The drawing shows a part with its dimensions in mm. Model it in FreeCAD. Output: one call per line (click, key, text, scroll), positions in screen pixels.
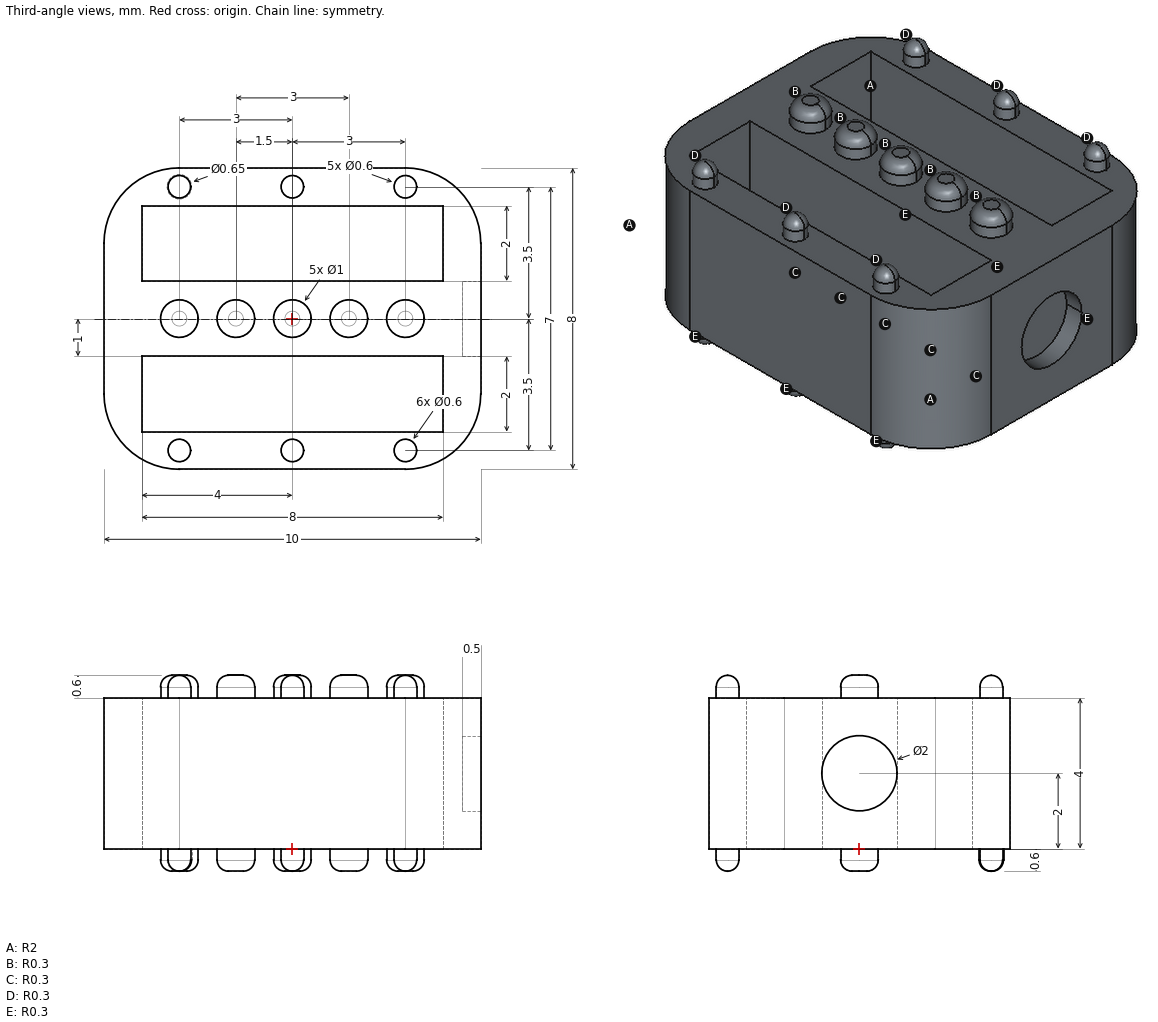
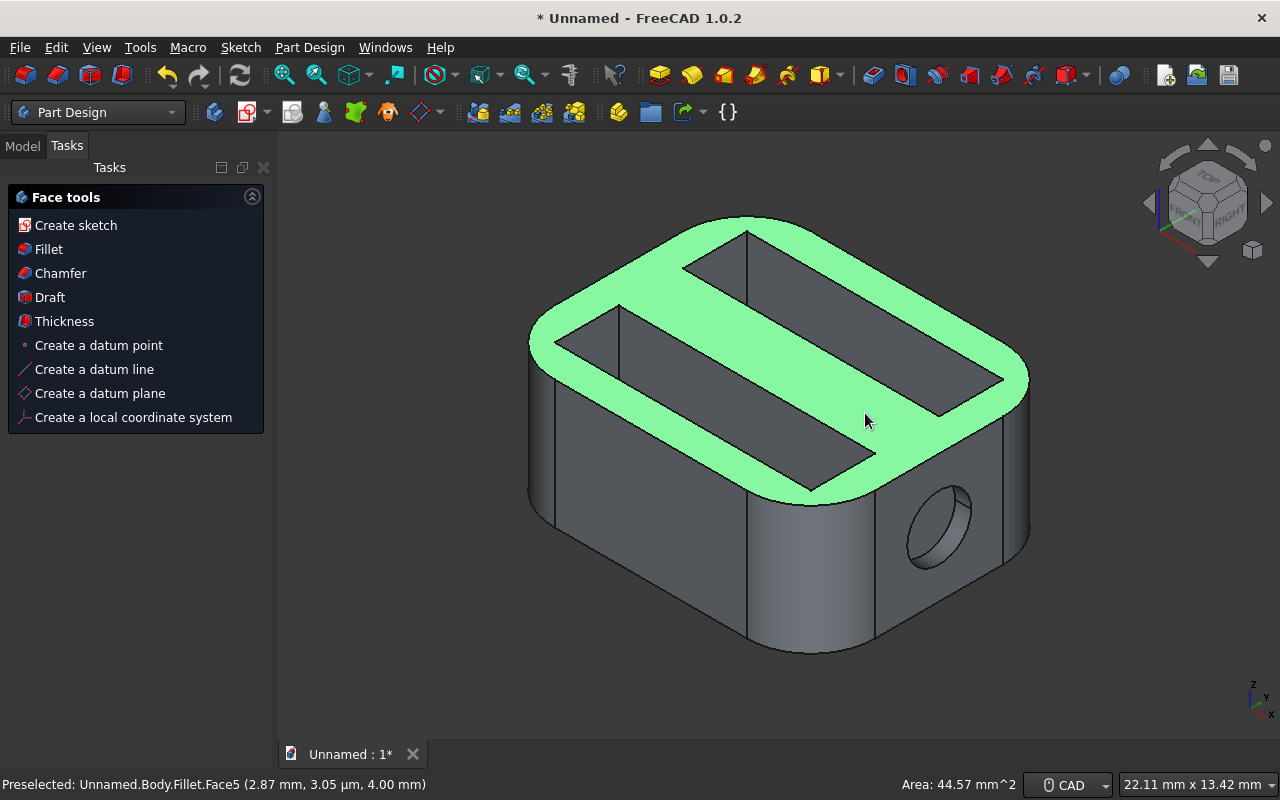
click(248, 112)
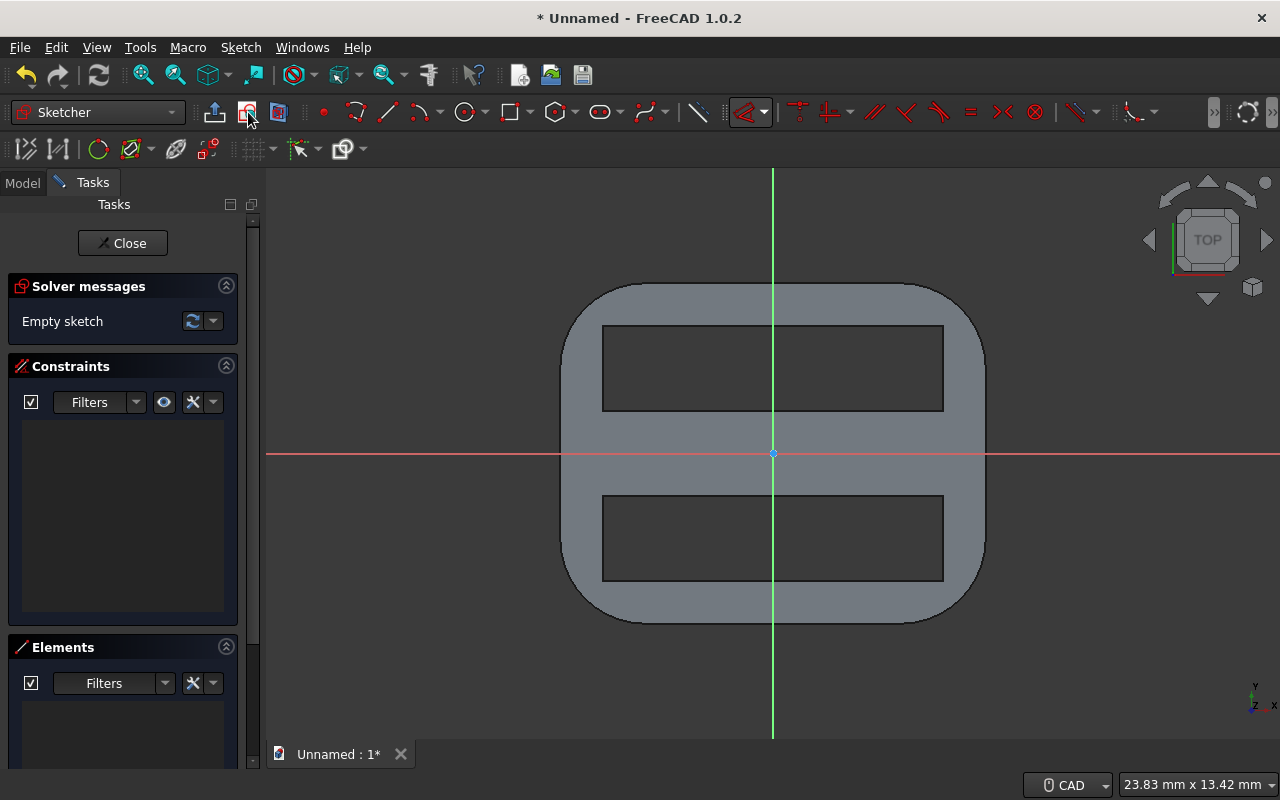
click(466, 112)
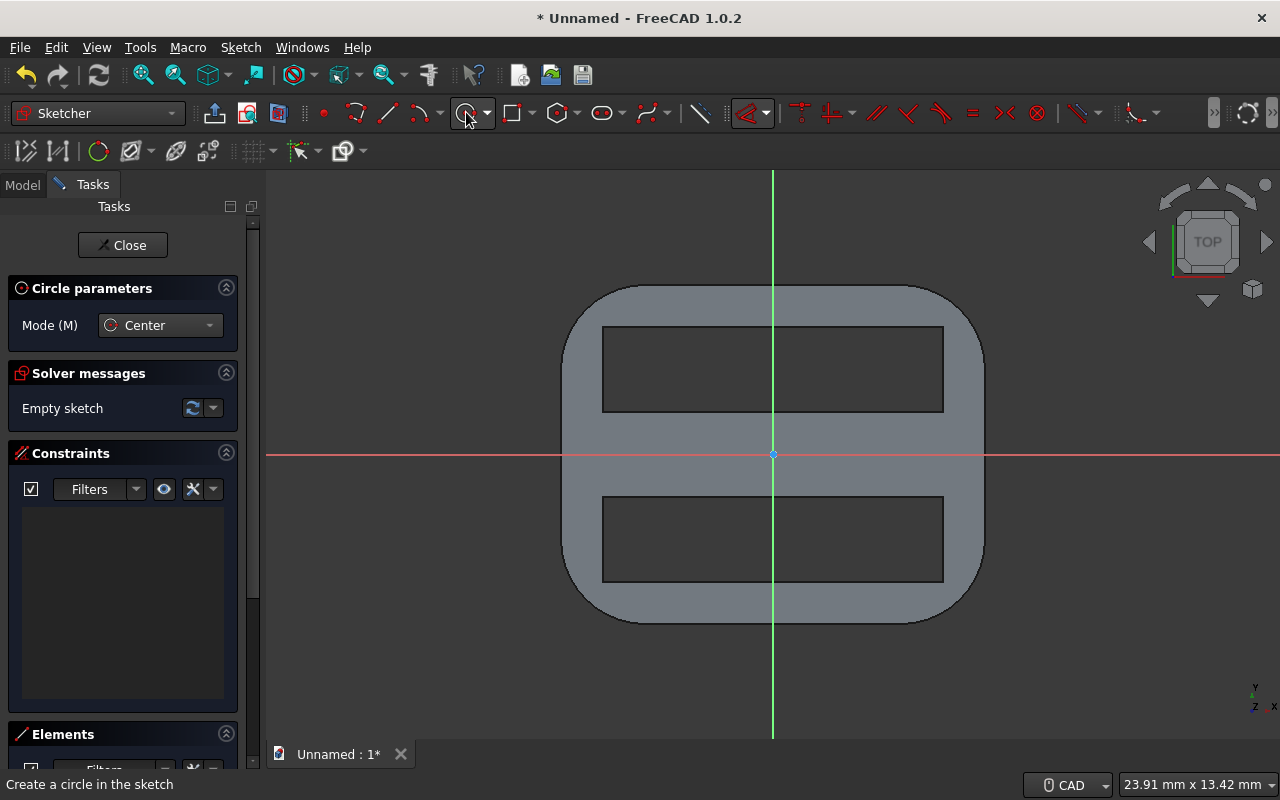
click(773, 455)
move(788, 440)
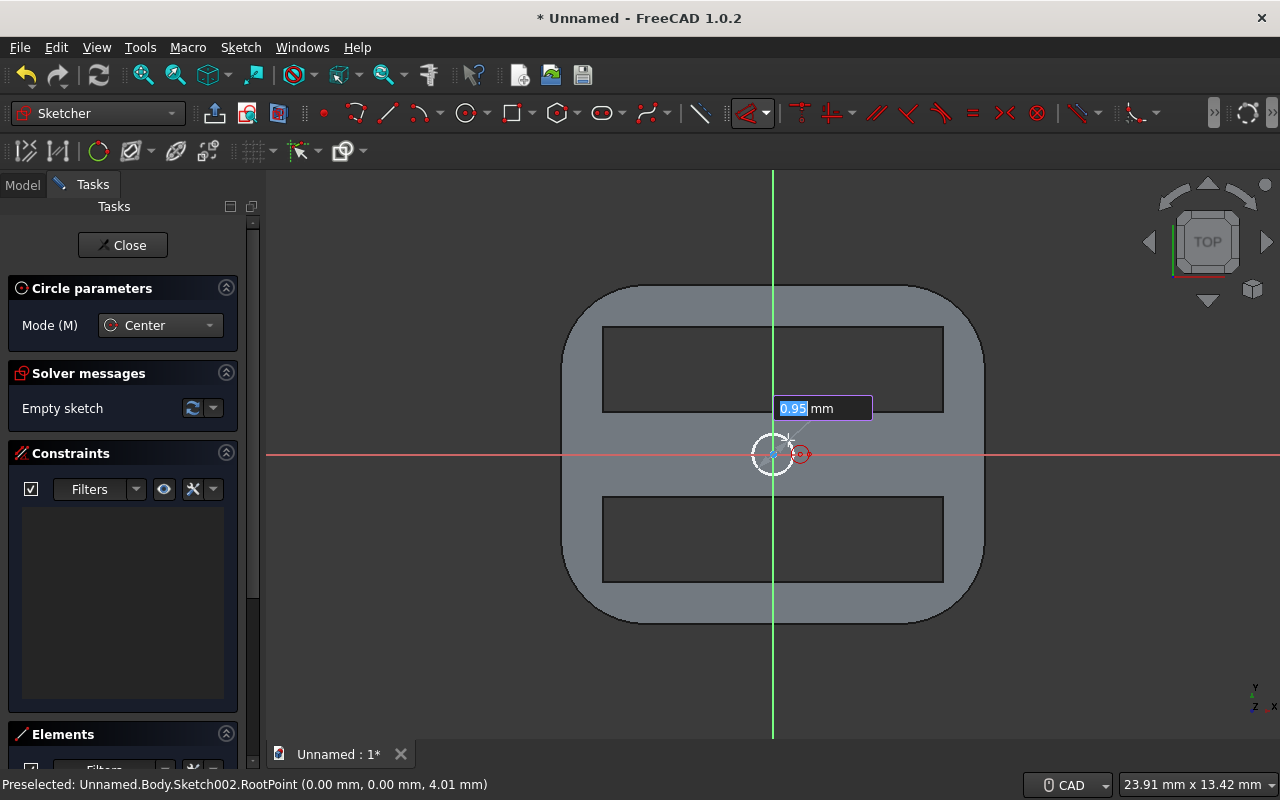
text(1)
key(Return)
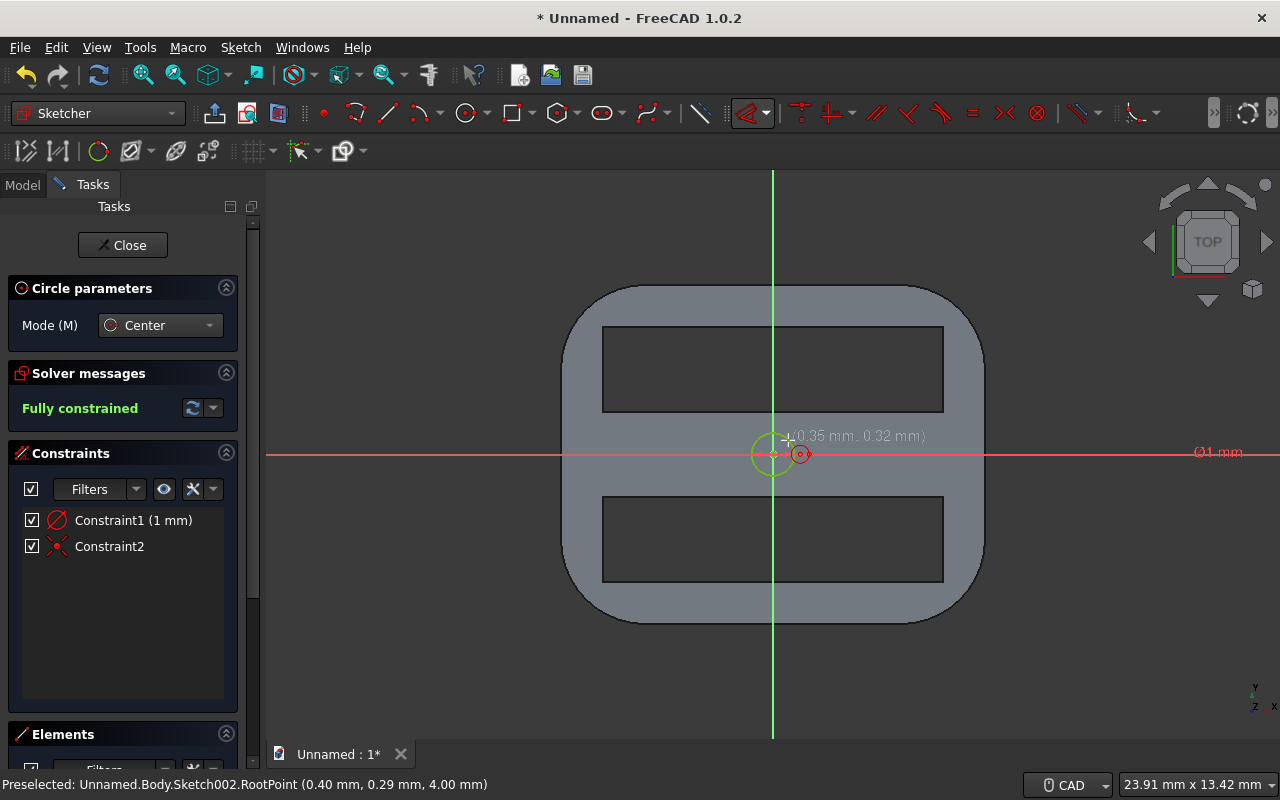
click(709, 455)
move(724, 440)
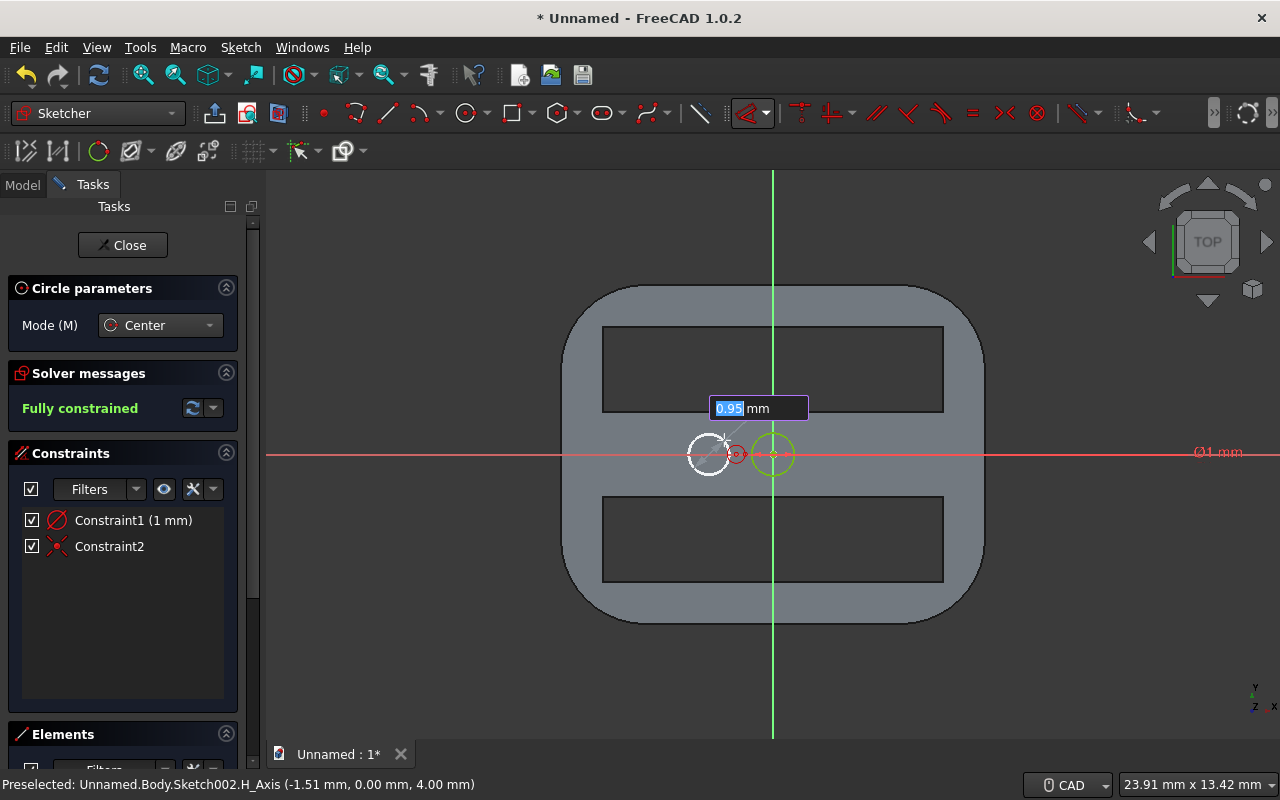
text(1)
key(Return)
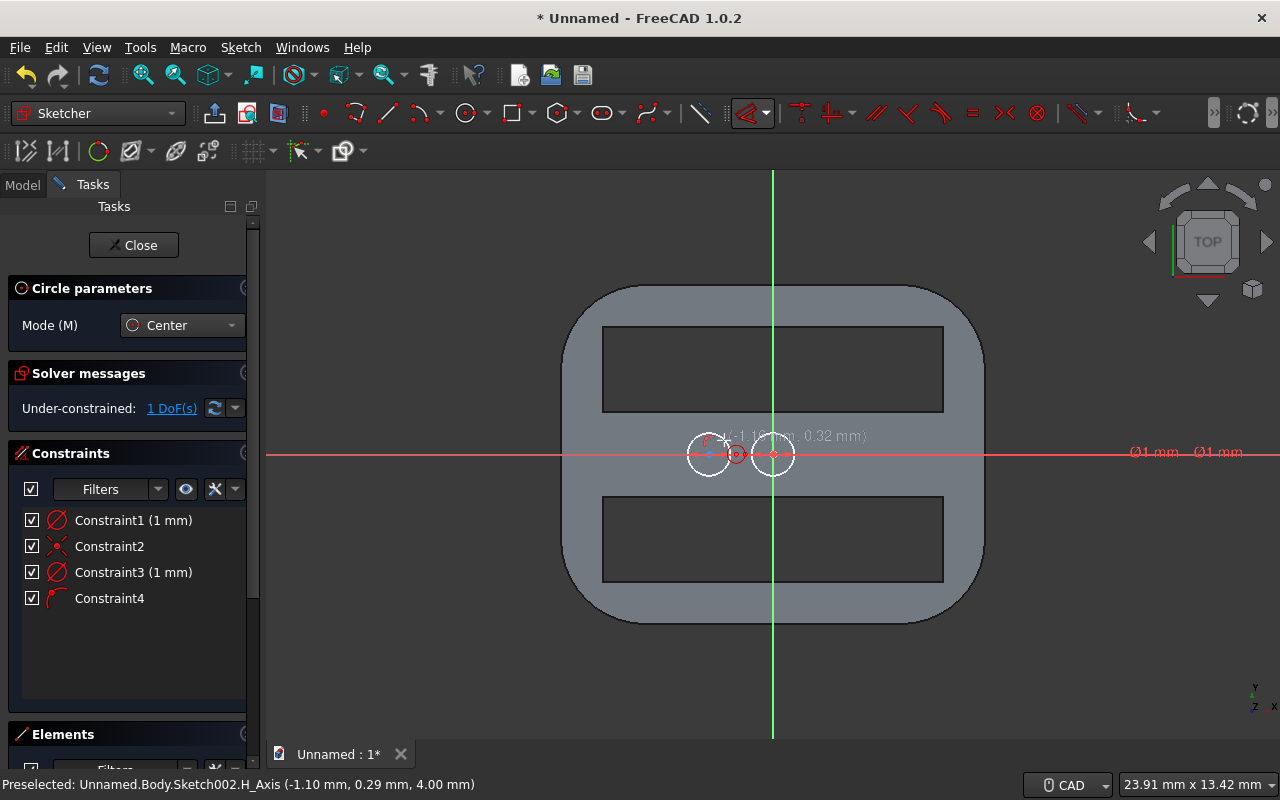
click(646, 455)
move(661, 440)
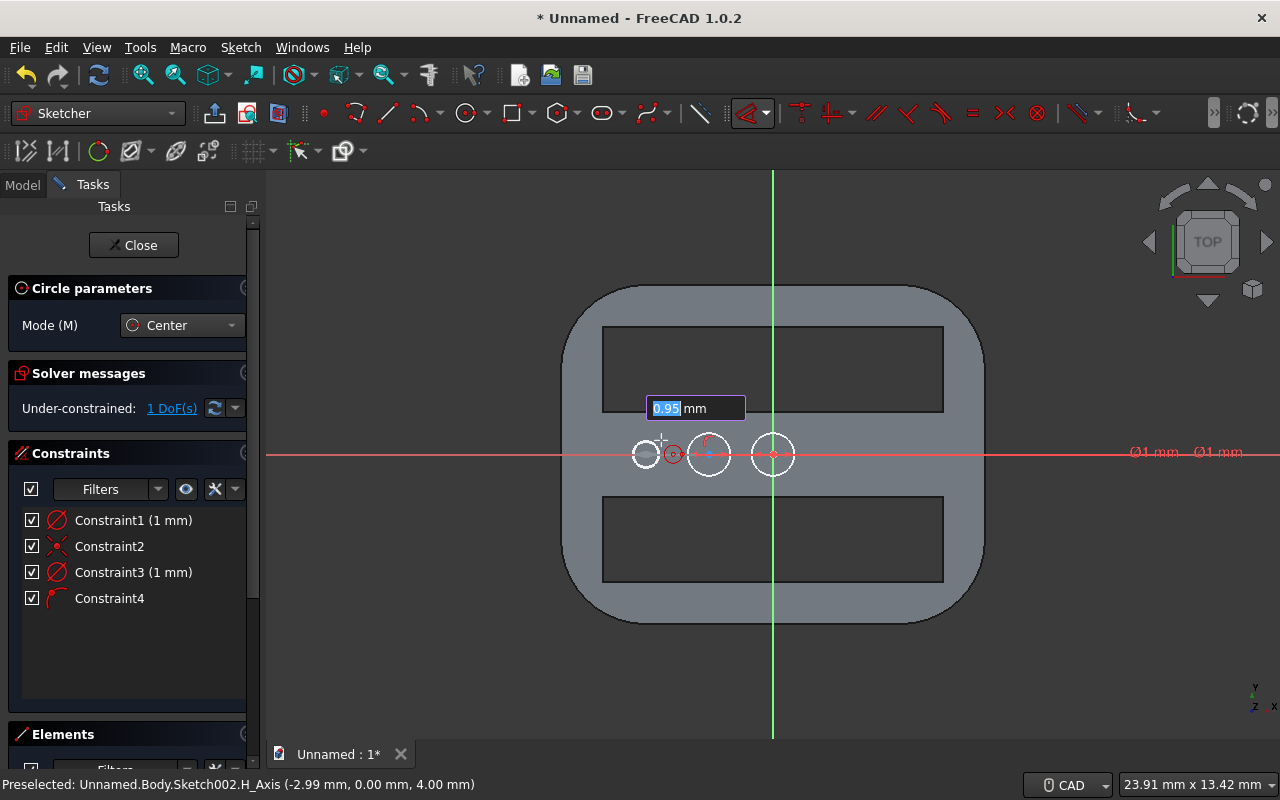
text(1)
key(Return)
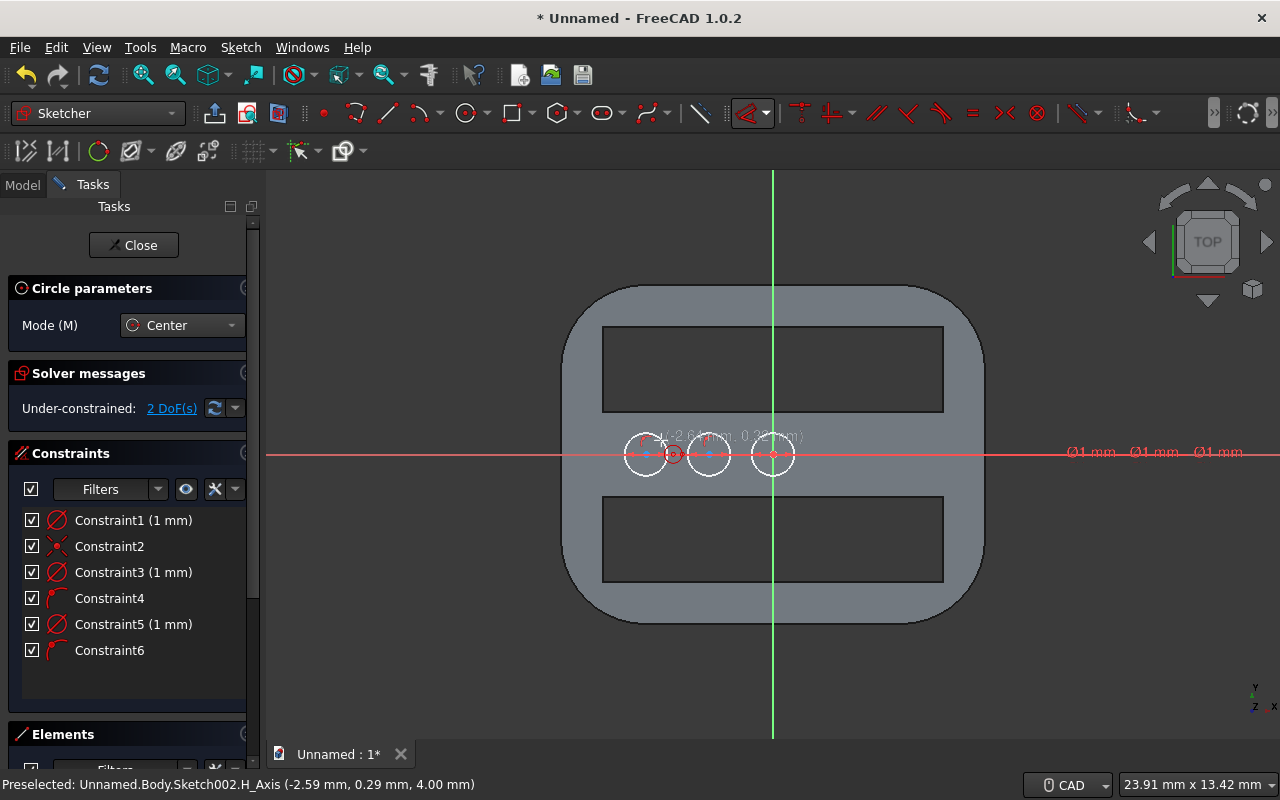
click(837, 455)
move(852, 440)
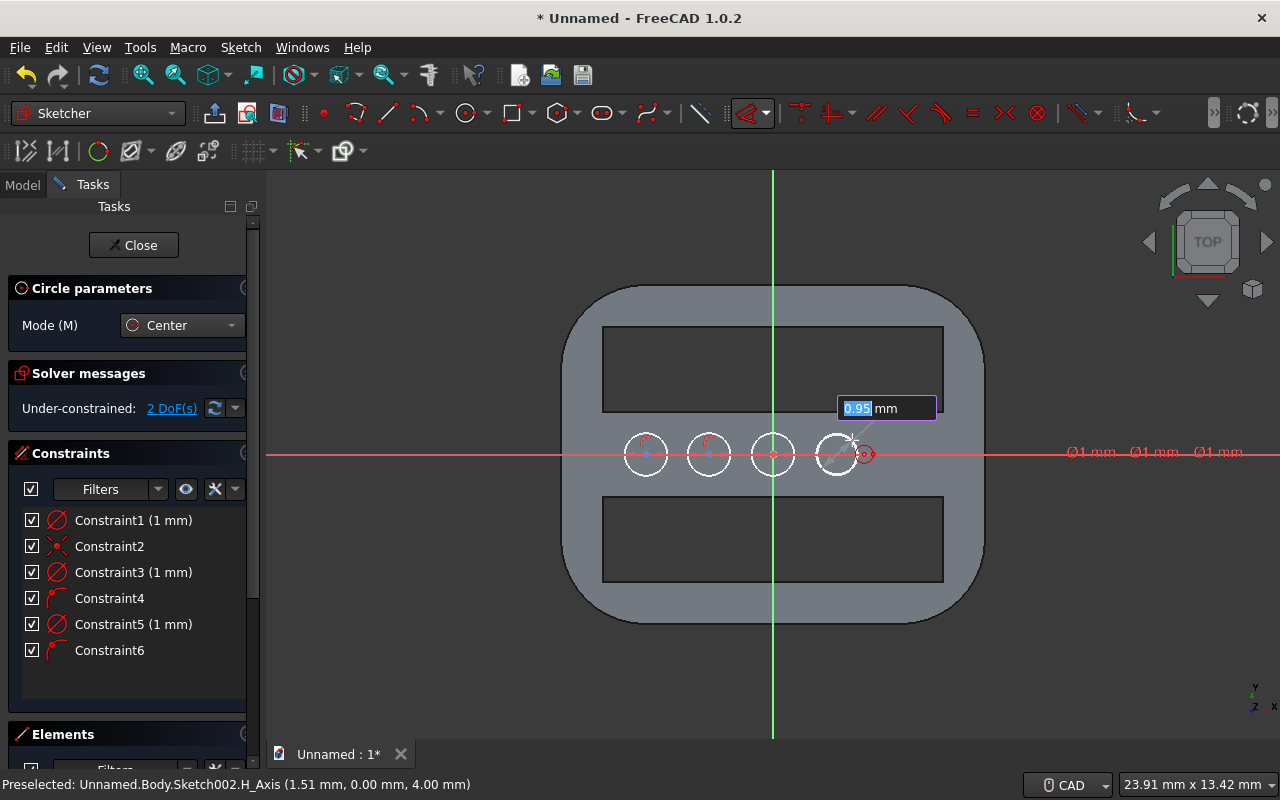
text(1)
key(Return)